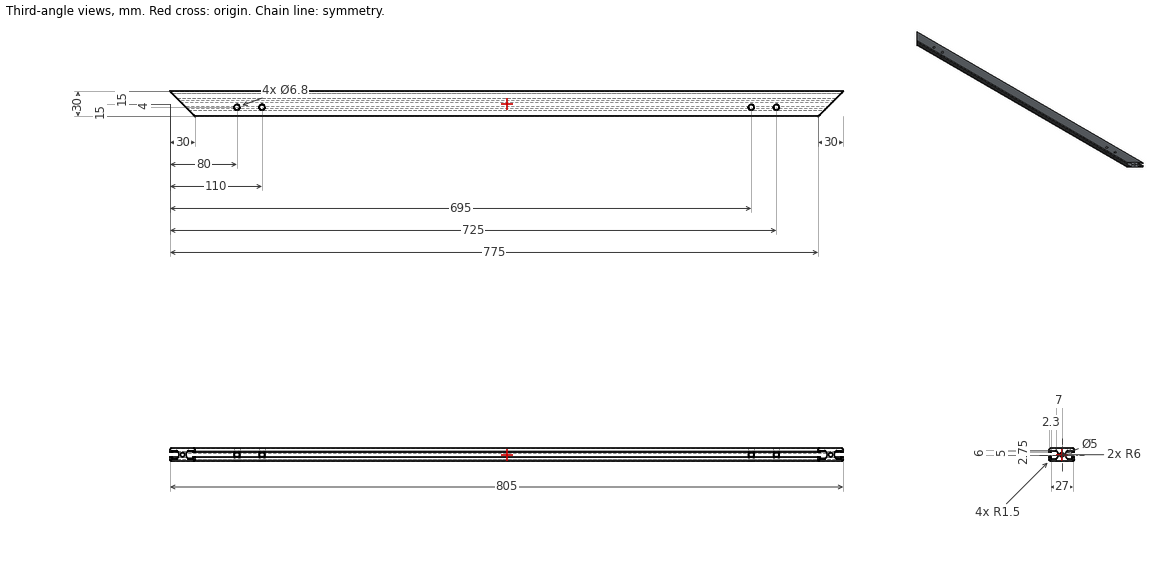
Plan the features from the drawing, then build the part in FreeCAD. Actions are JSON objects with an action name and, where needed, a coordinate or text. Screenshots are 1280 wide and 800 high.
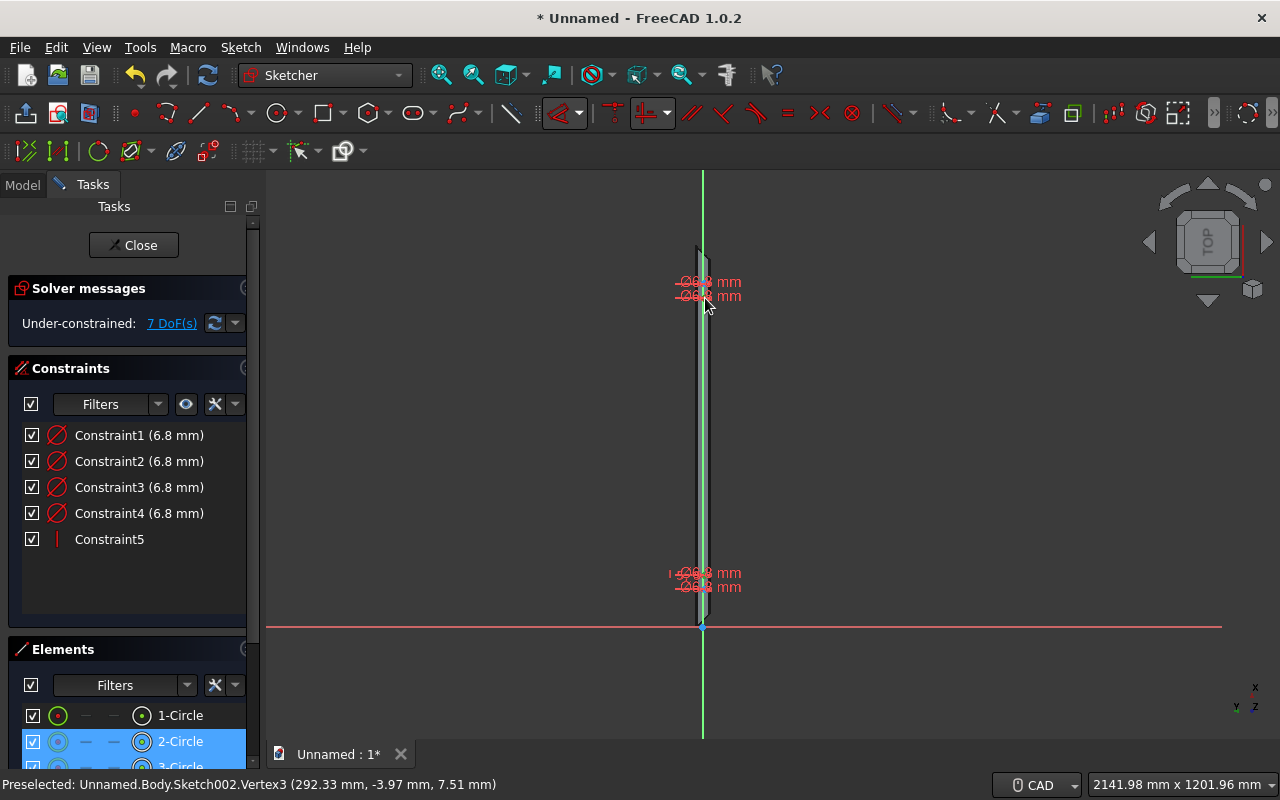
{"action": "key", "text": "v"}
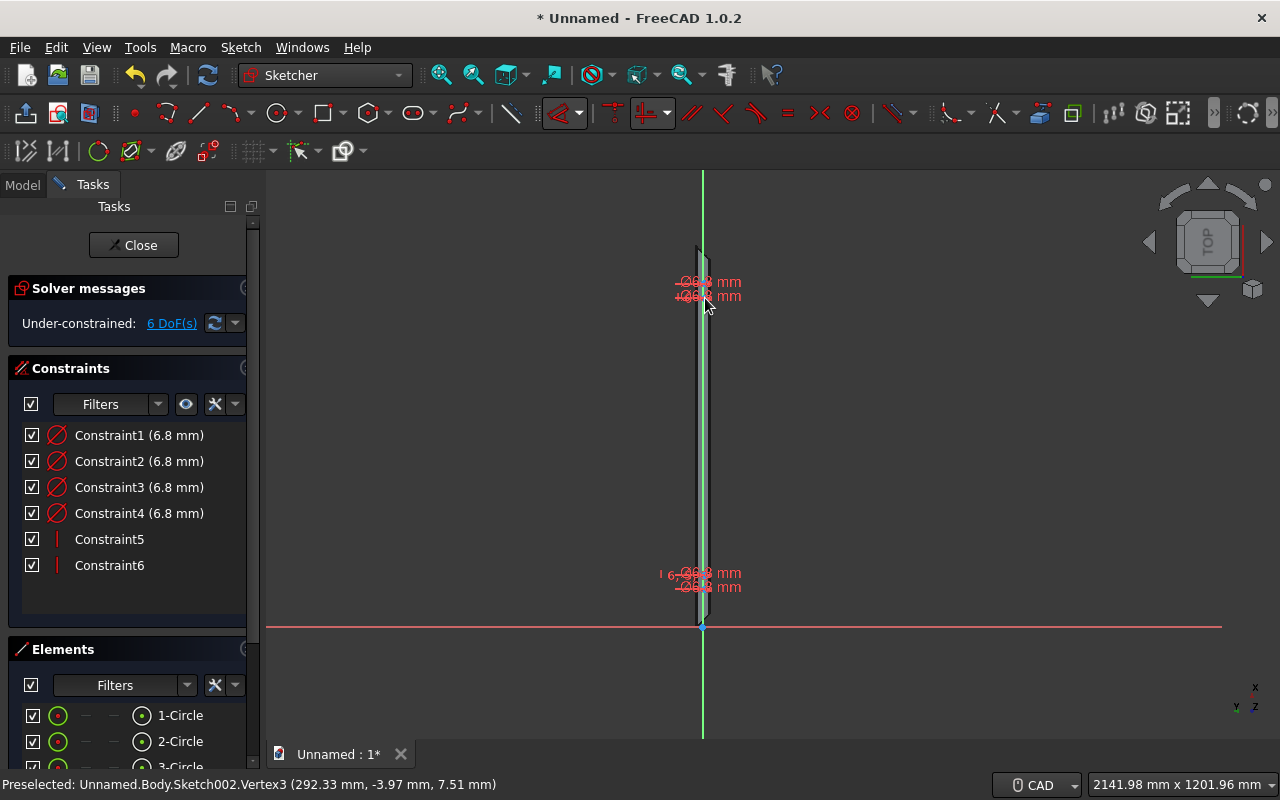
{"action": "left_click", "coordinate": [705, 298]}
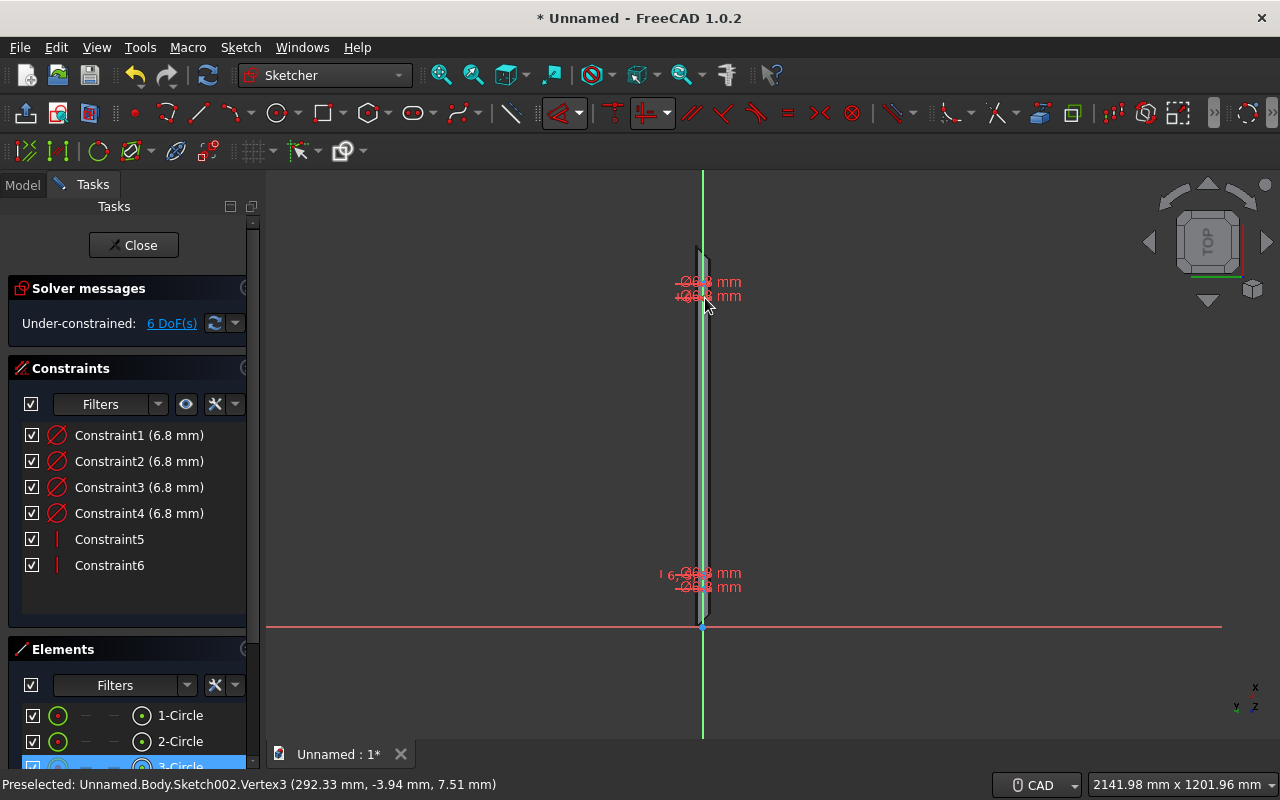
{"action": "left_click", "coordinate": [705, 284]}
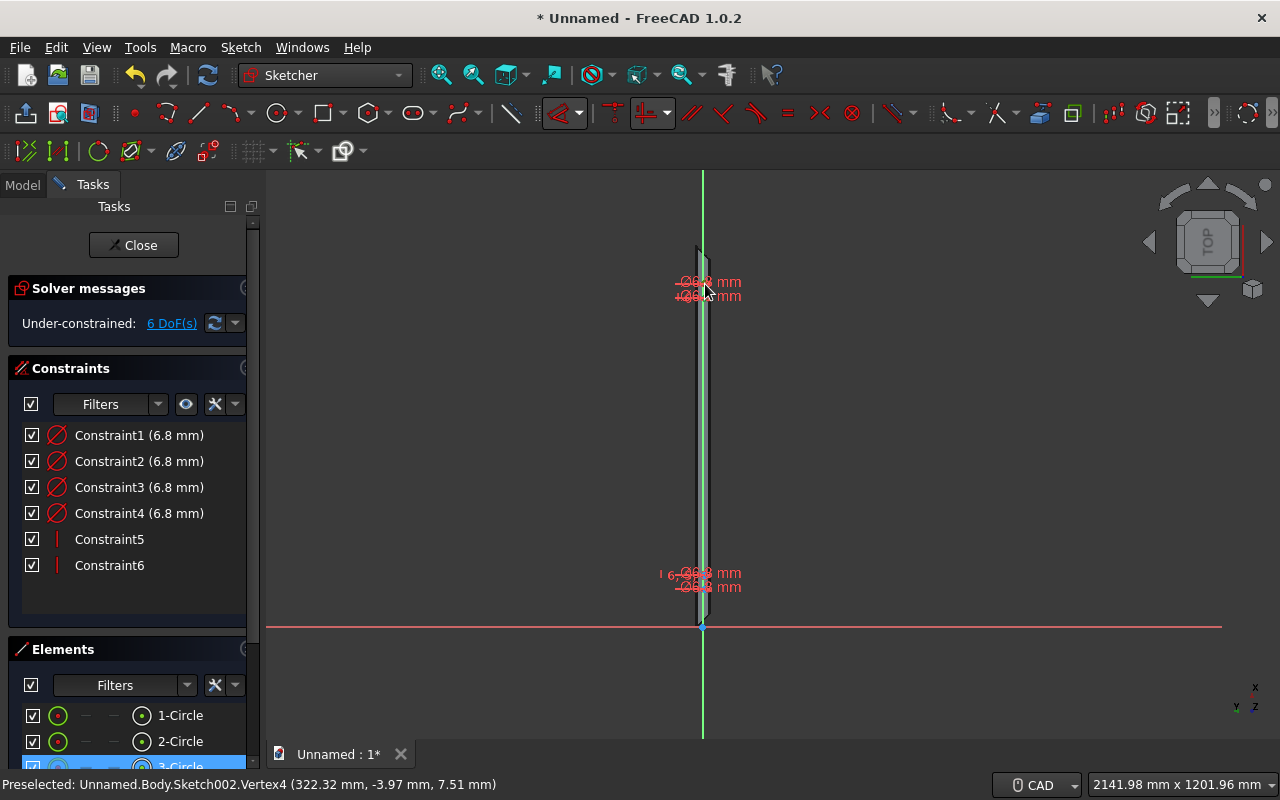
{"action": "key", "text": "v"}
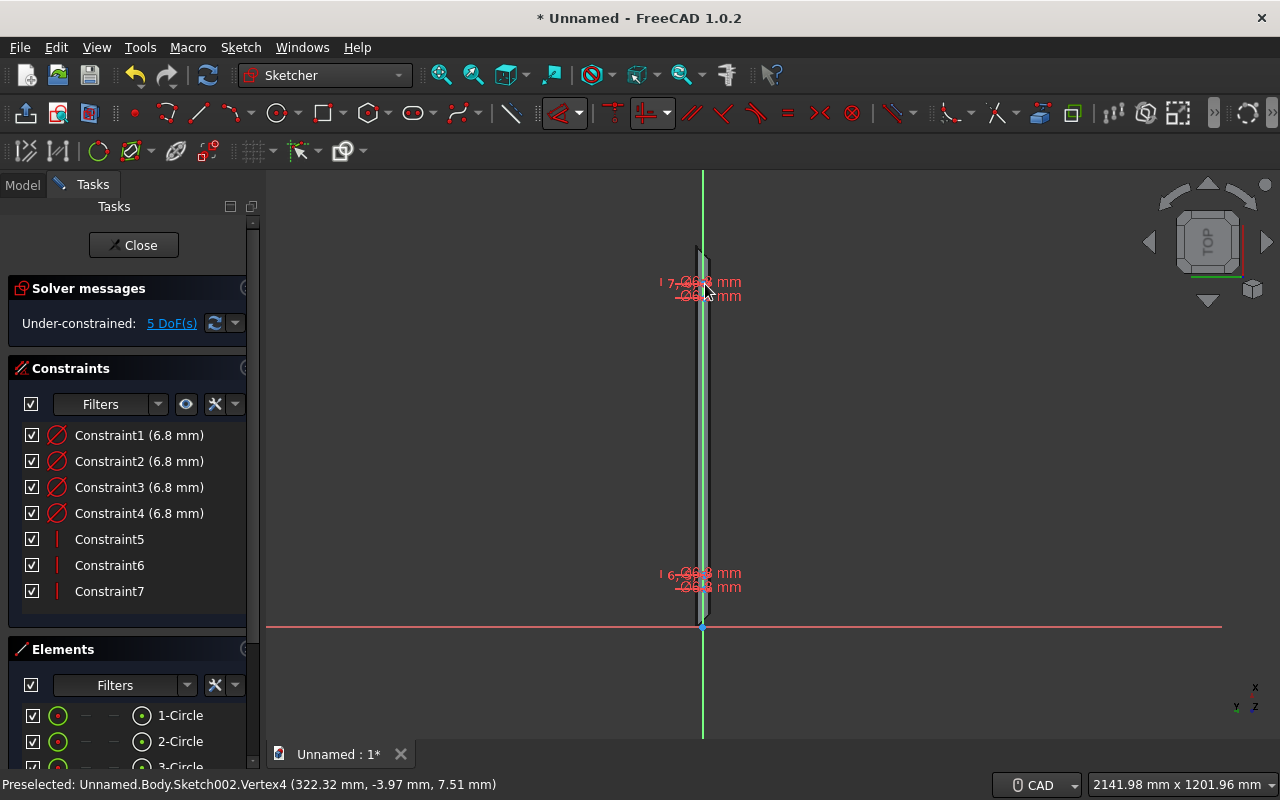
{"action": "scroll", "coordinate": [705, 589], "scroll_direction": "up", "scroll_amount": 16}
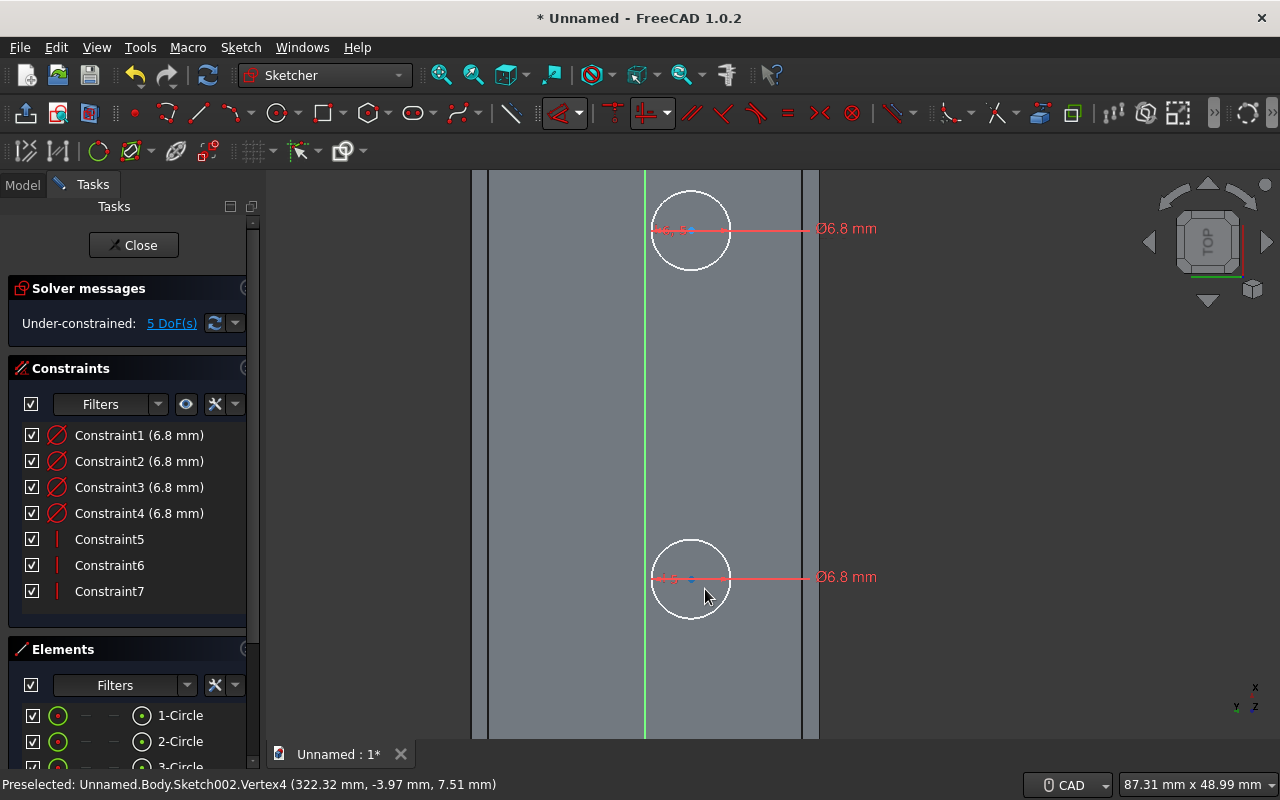
{"action": "left_click", "coordinate": [691, 579]}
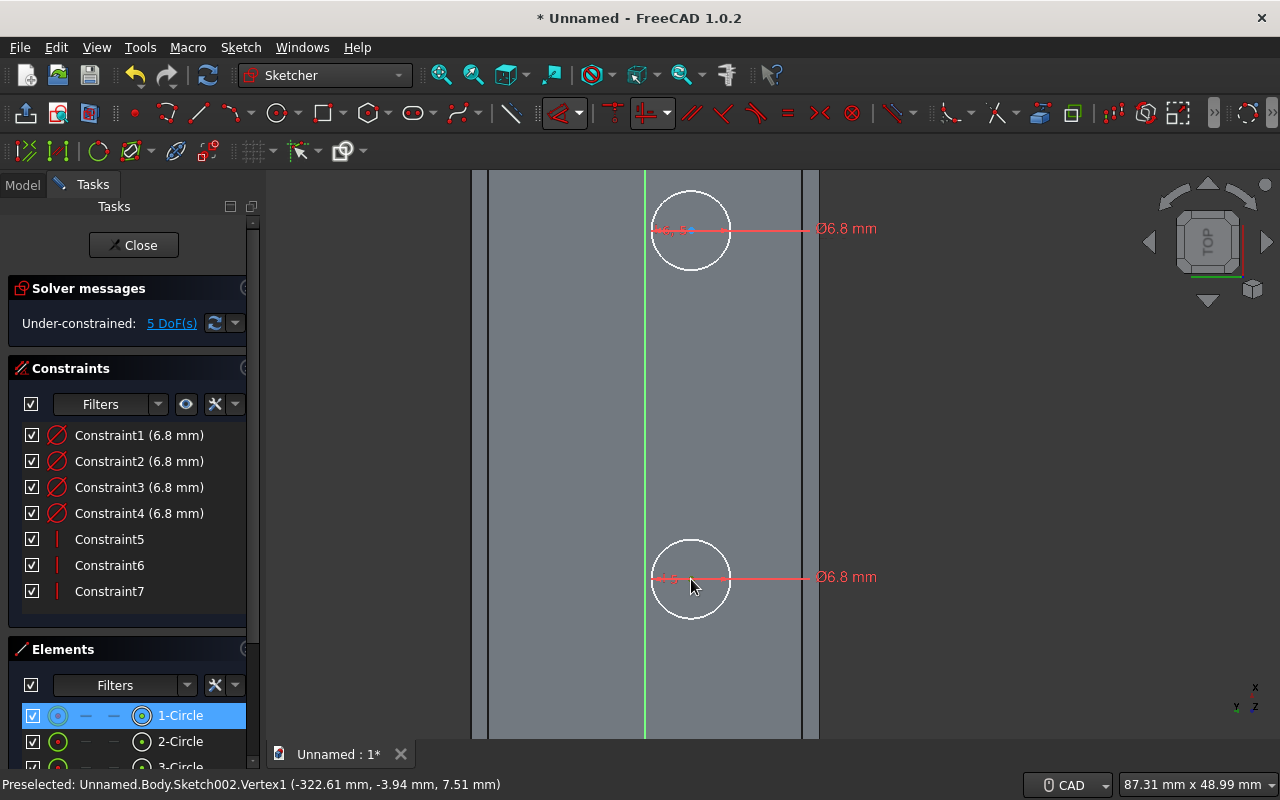
{"action": "left_click", "coordinate": [582, 114]}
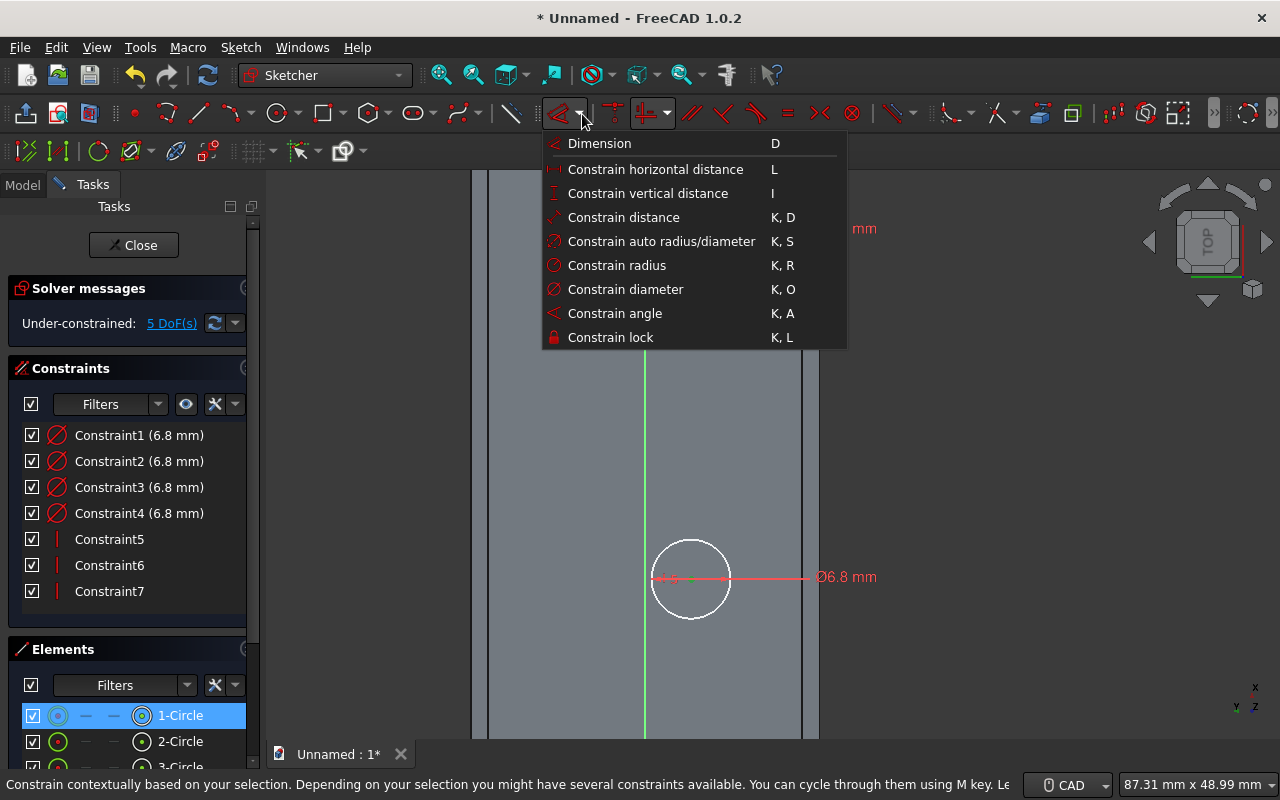
{"action": "left_click", "coordinate": [695, 169]}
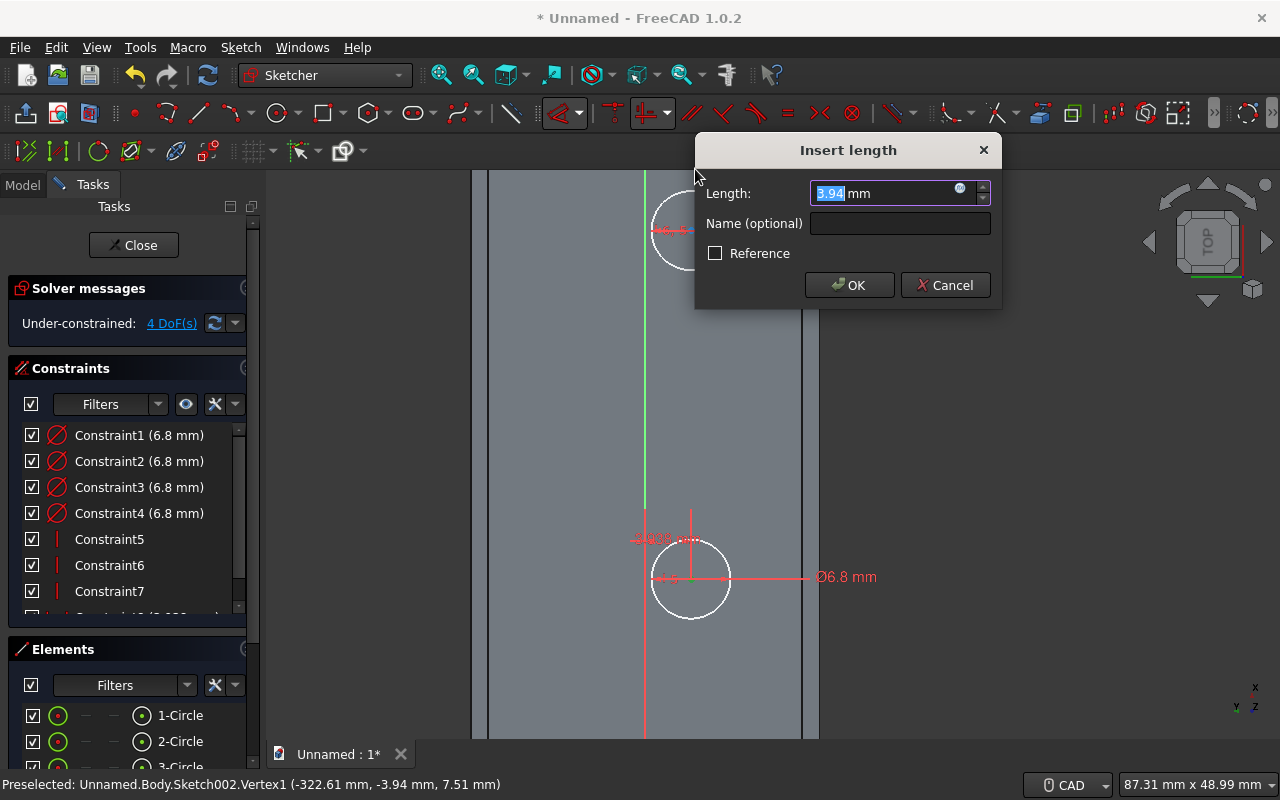
{"action": "type", "text": "4"}
{"action": "key", "text": "Return"}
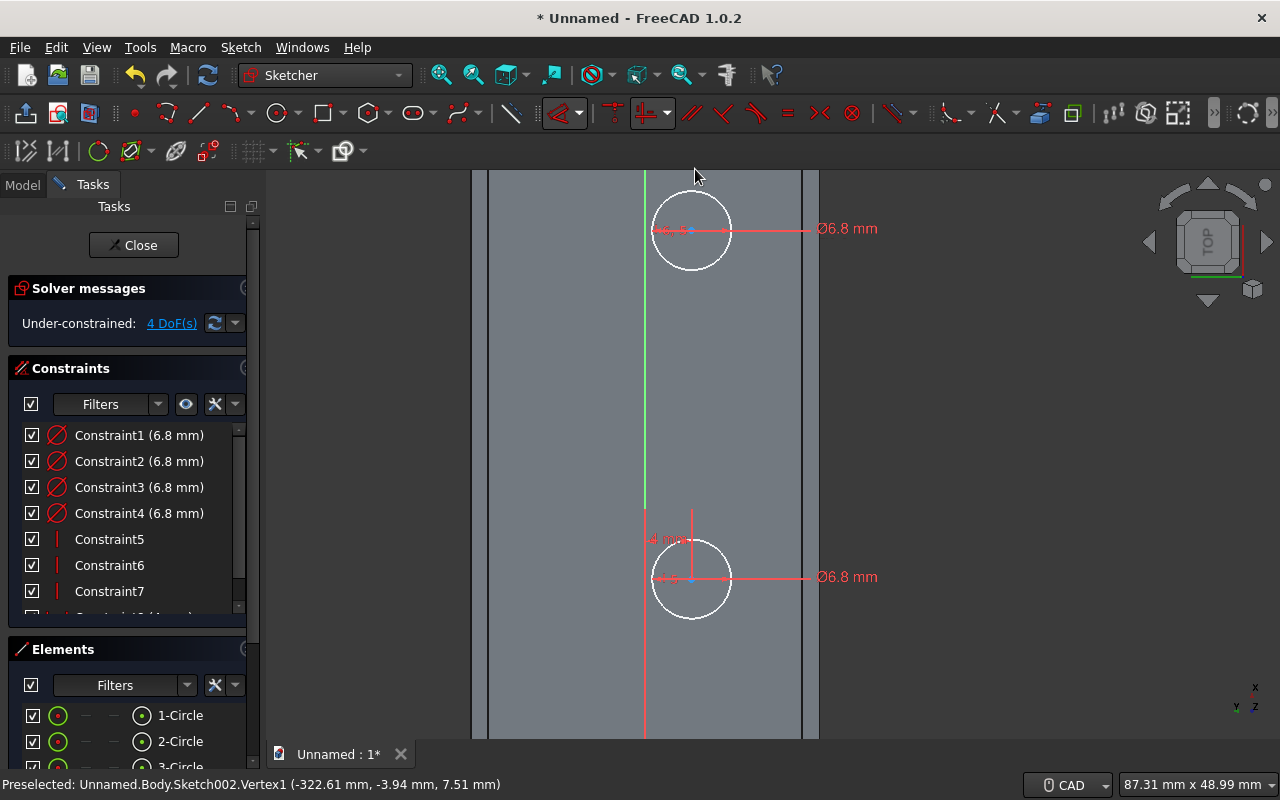
{"action": "scroll", "coordinate": [705, 621], "scroll_direction": "down", "scroll_amount": 15}